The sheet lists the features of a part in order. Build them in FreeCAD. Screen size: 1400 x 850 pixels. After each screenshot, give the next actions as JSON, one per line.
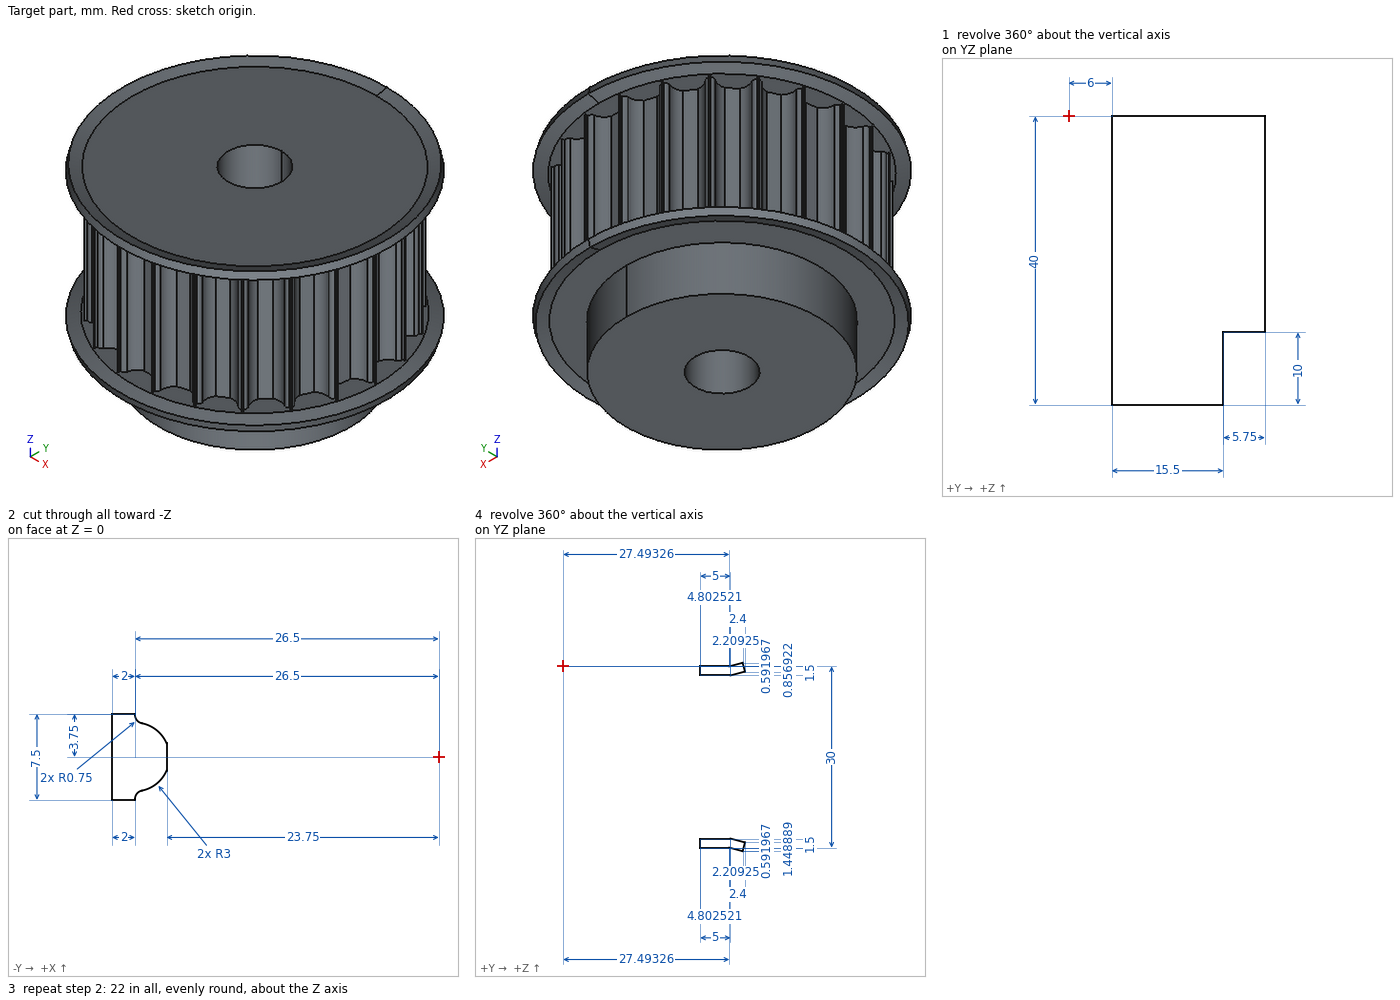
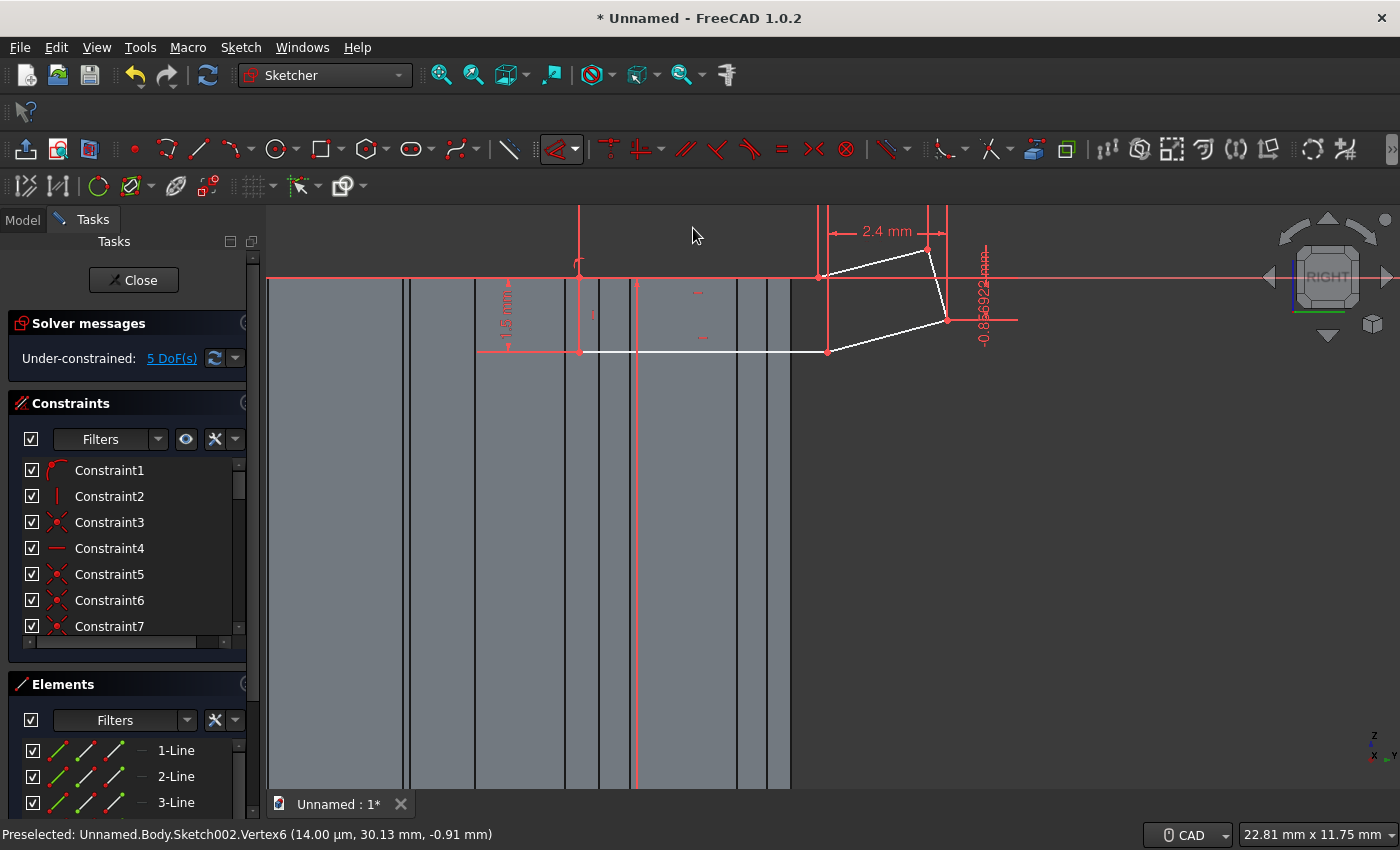
{"action": "scroll", "coordinate": [928, 250], "scroll_direction": "up", "scroll_amount": 2}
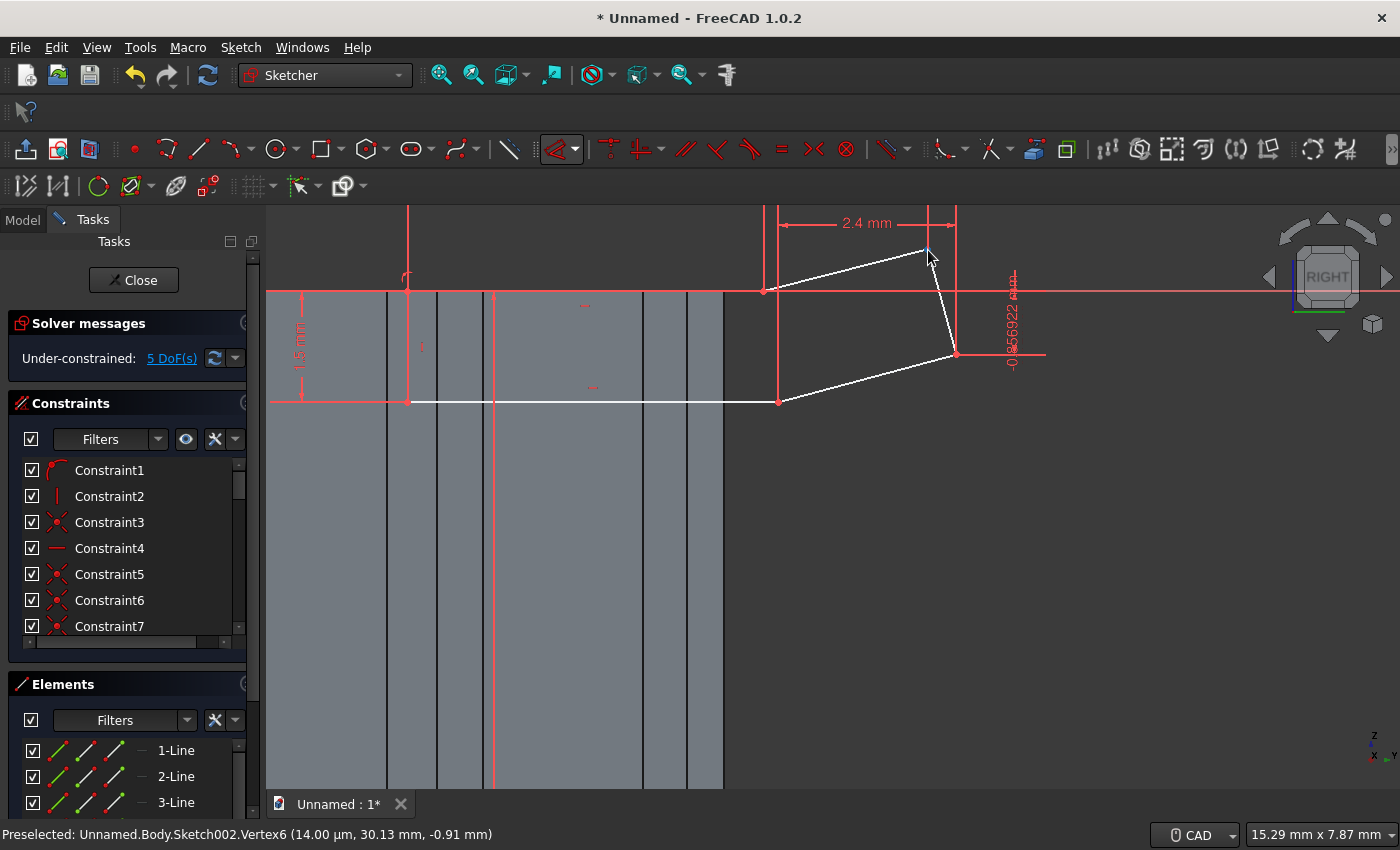
{"action": "left_click", "coordinate": [928, 249]}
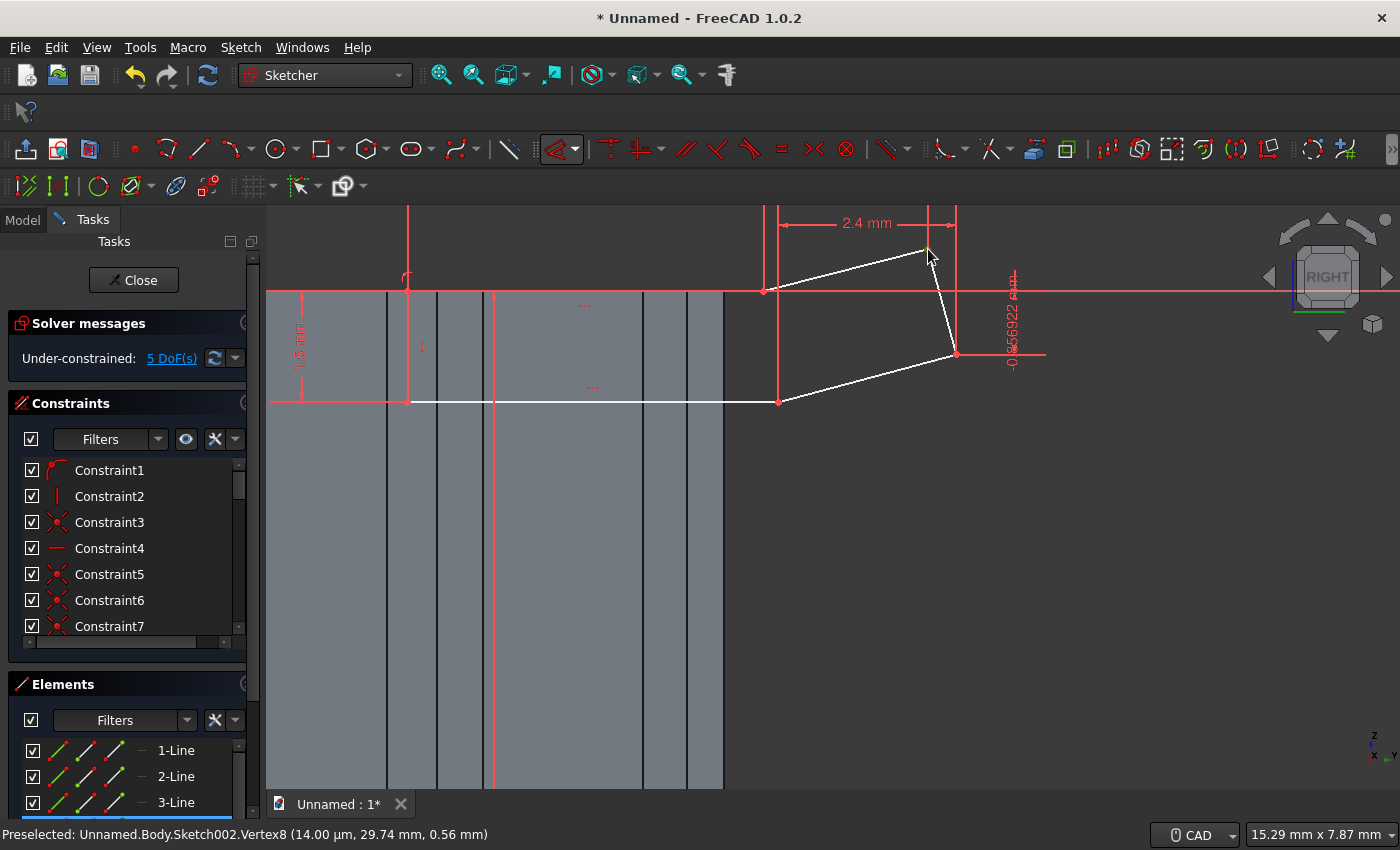
{"action": "key", "text": "i"}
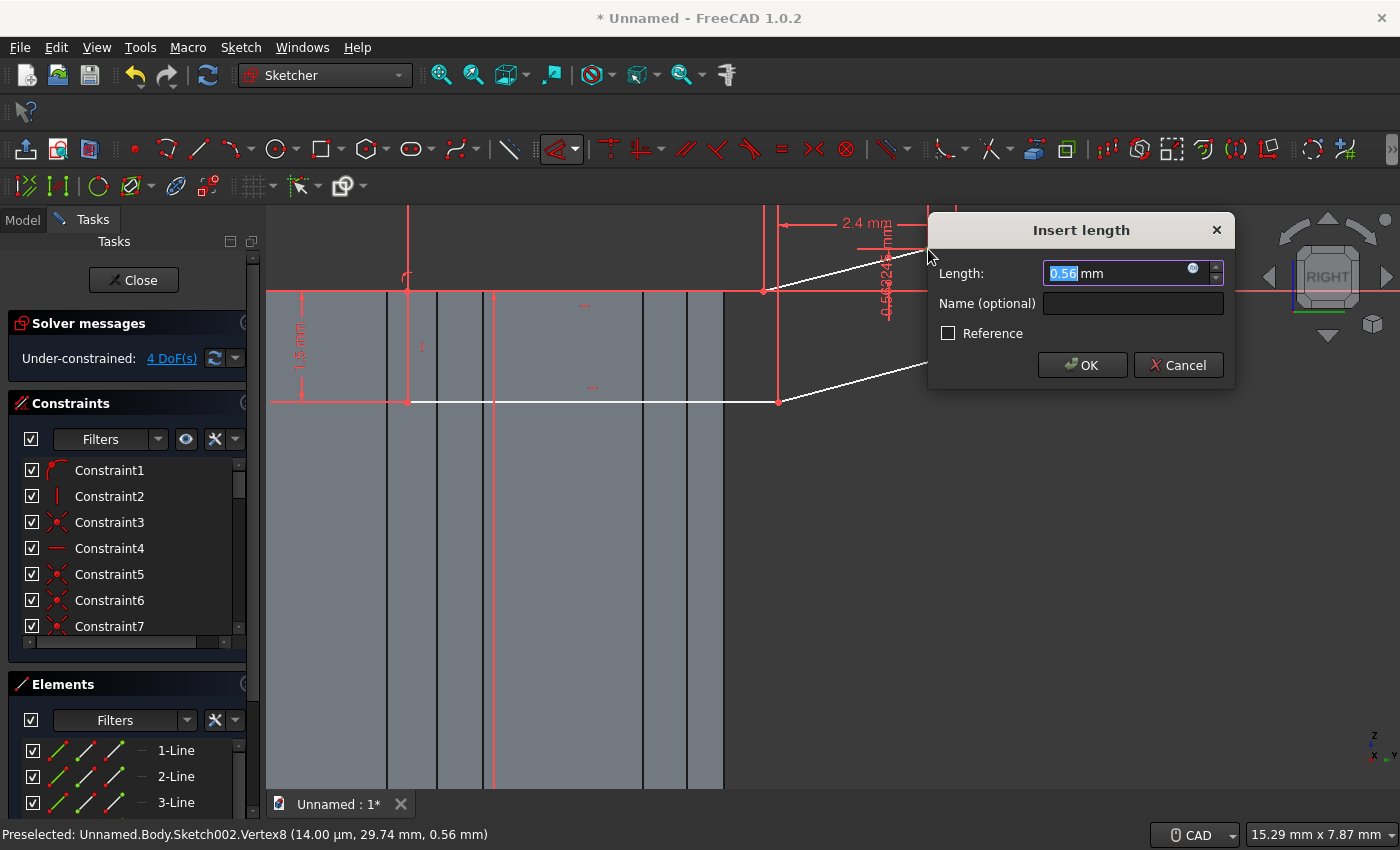
{"action": "type", "text": "0.591967"}
{"action": "key", "text": "Return"}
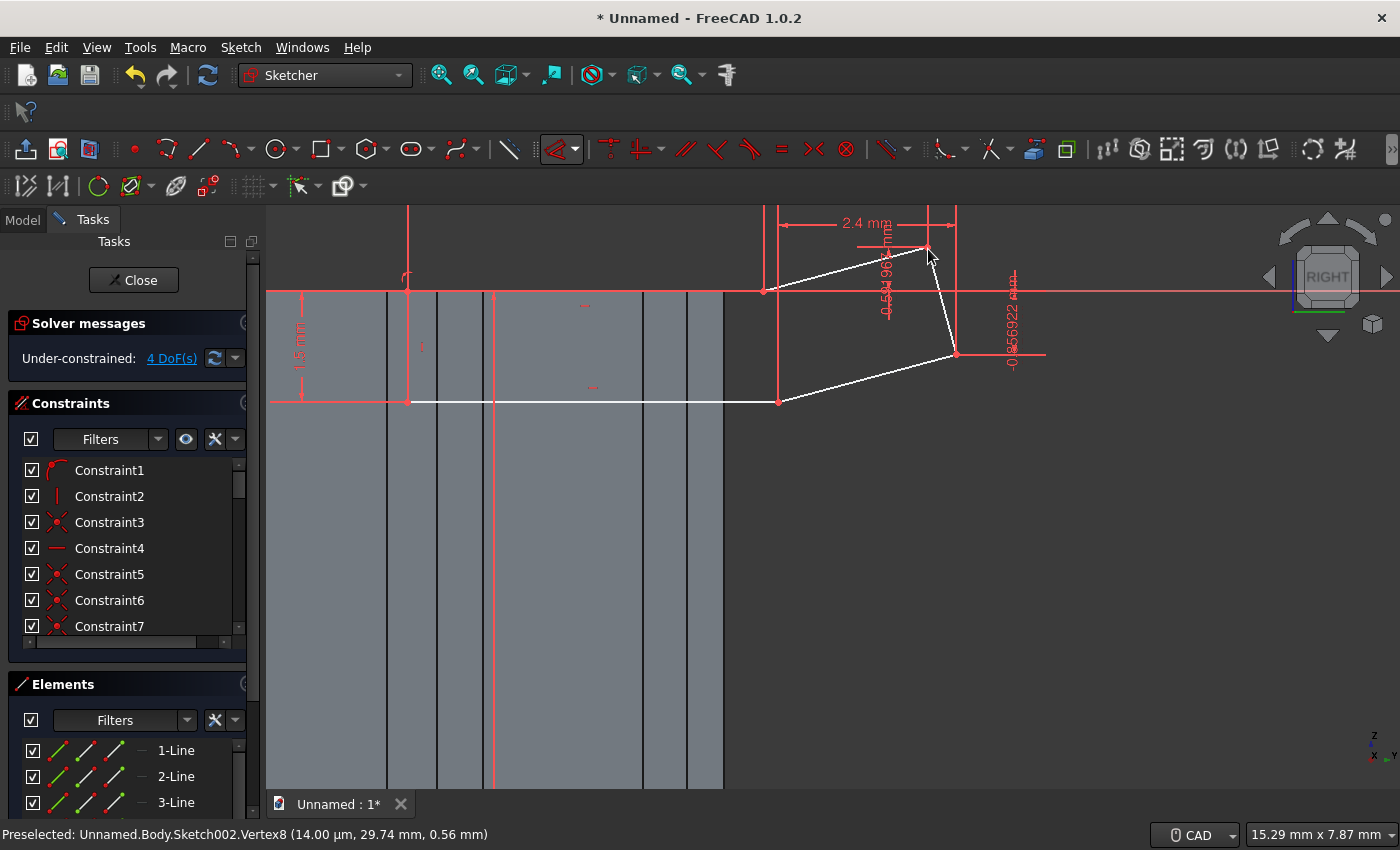
{"action": "scroll", "coordinate": [948, 317], "scroll_direction": "down", "scroll_amount": 9}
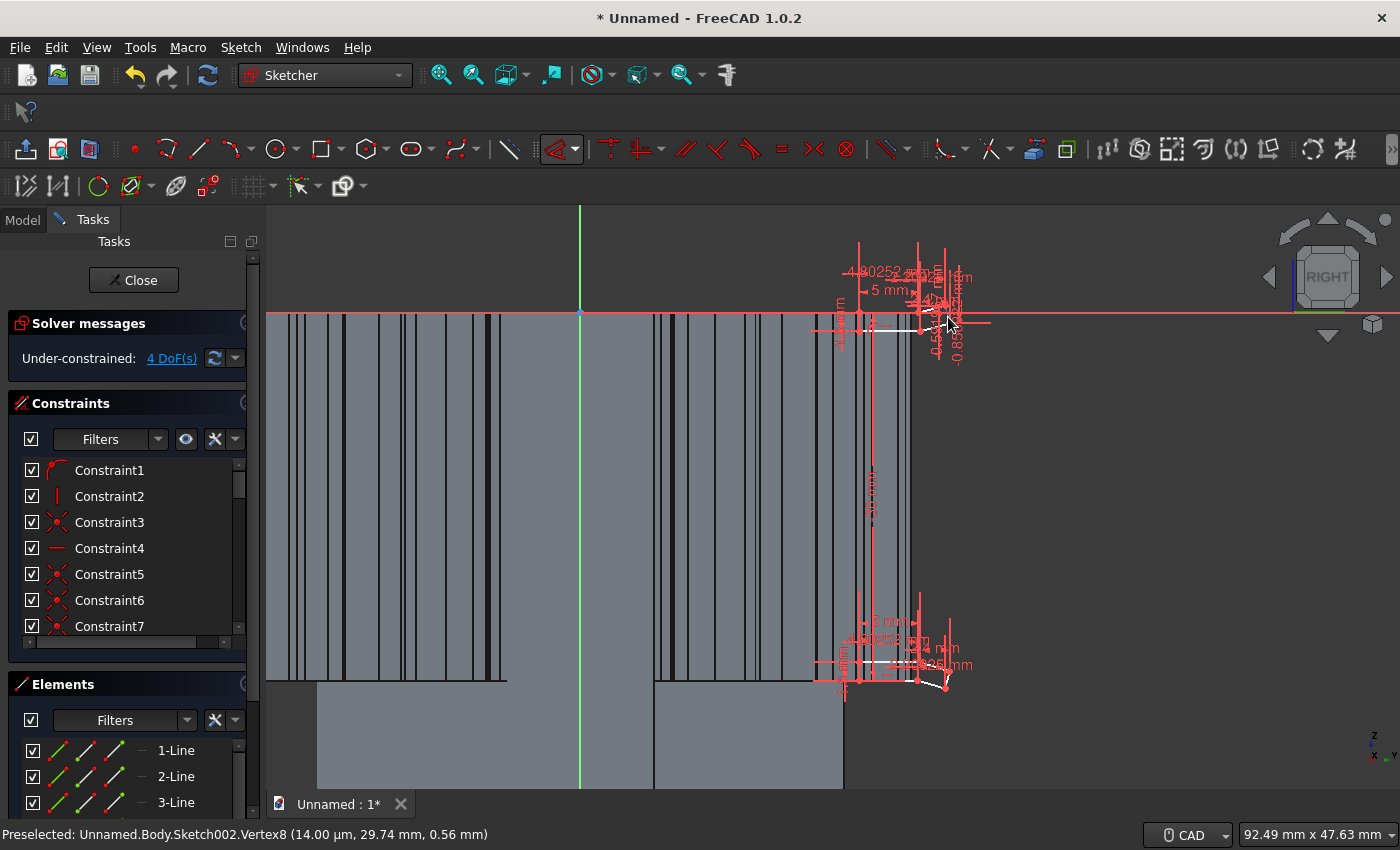
{"action": "left_click", "coordinate": [918, 313]}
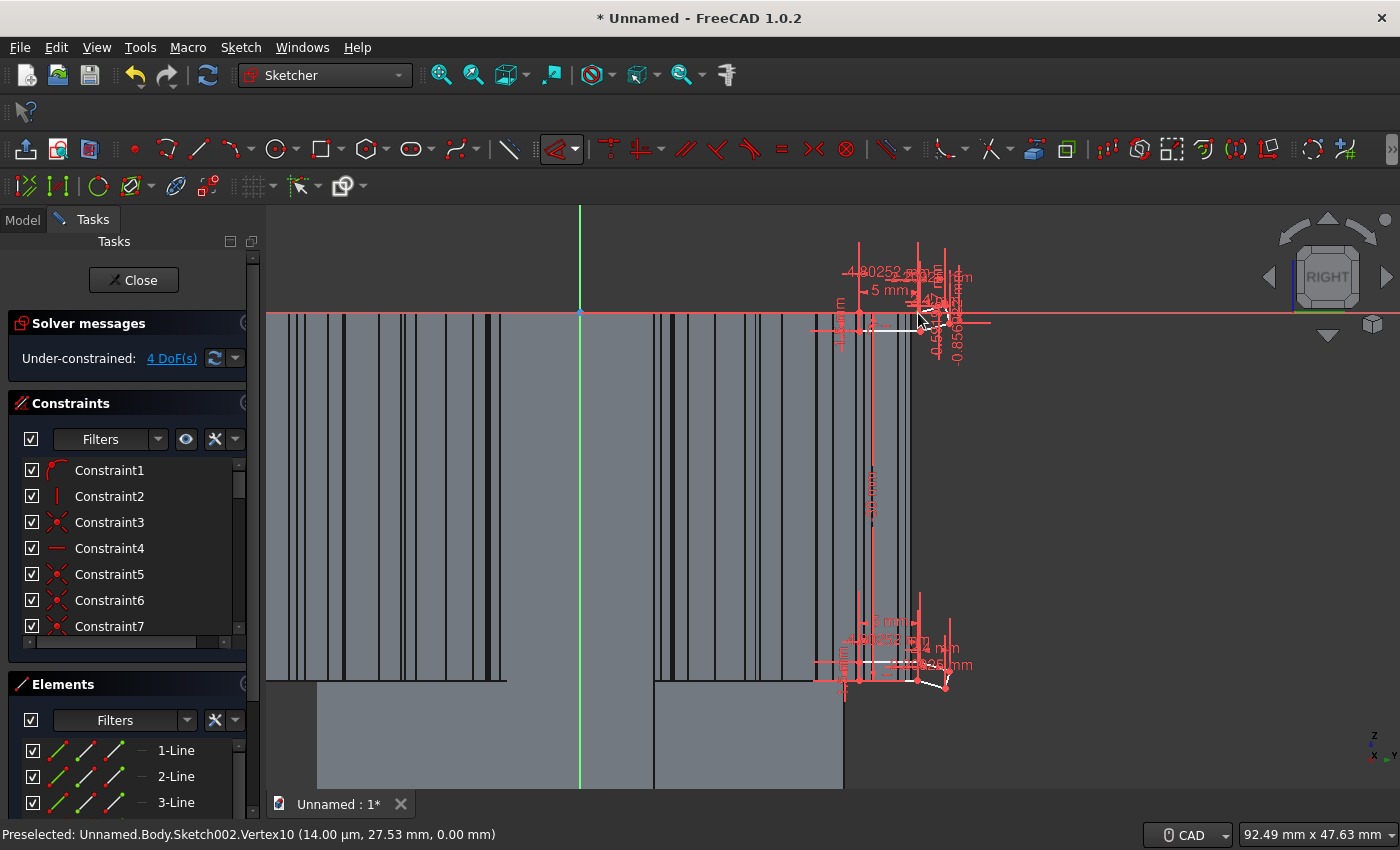
{"action": "left_click", "coordinate": [578, 150]}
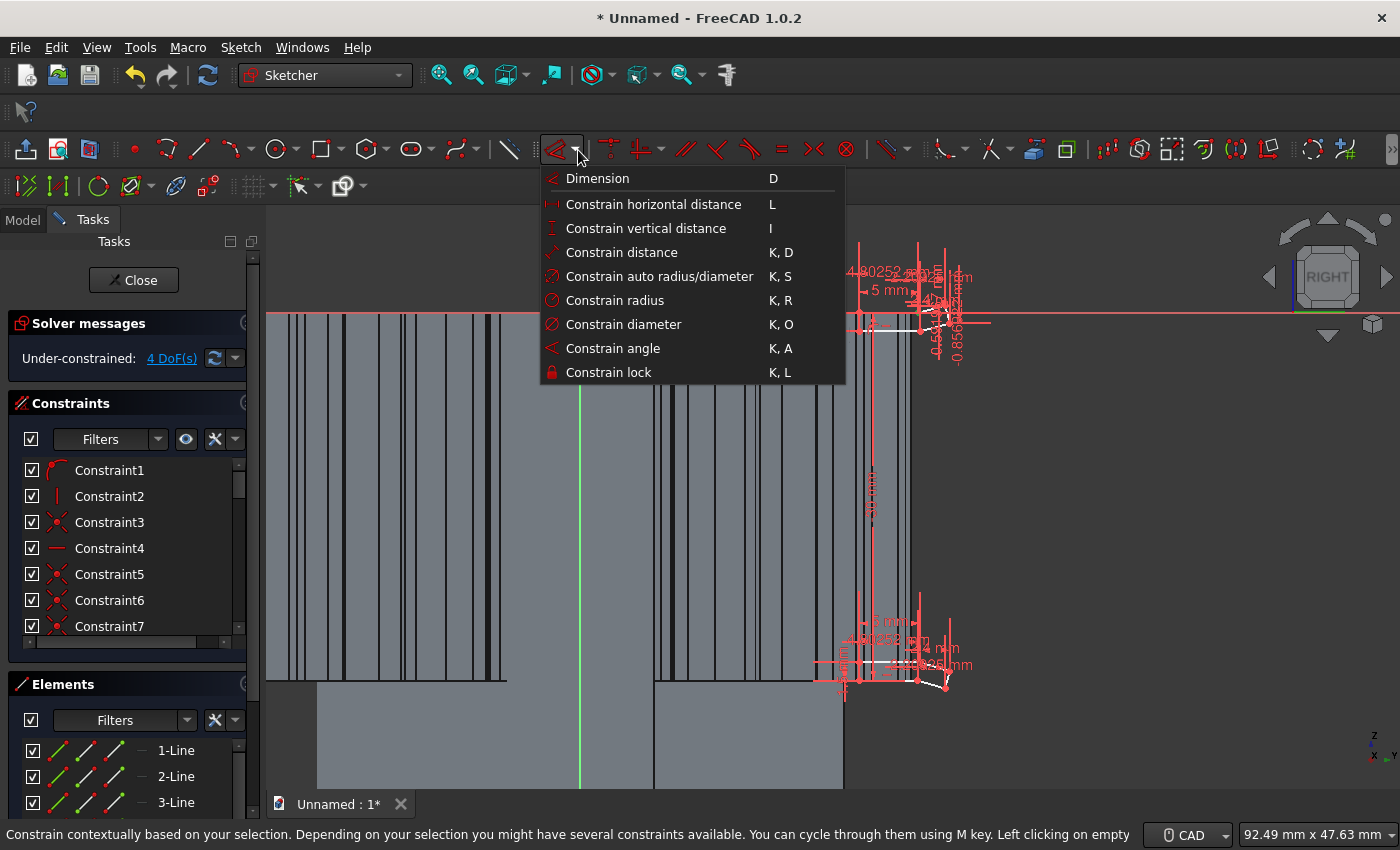
{"action": "left_click", "coordinate": [693, 204]}